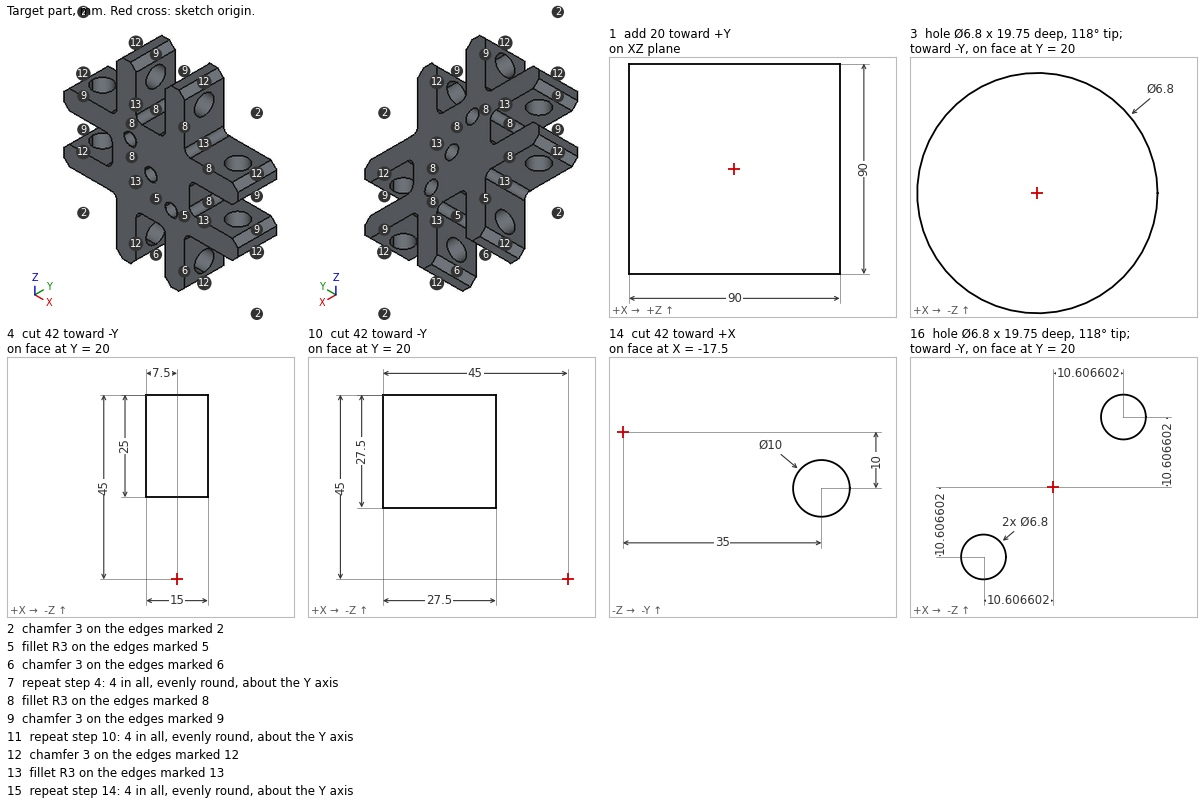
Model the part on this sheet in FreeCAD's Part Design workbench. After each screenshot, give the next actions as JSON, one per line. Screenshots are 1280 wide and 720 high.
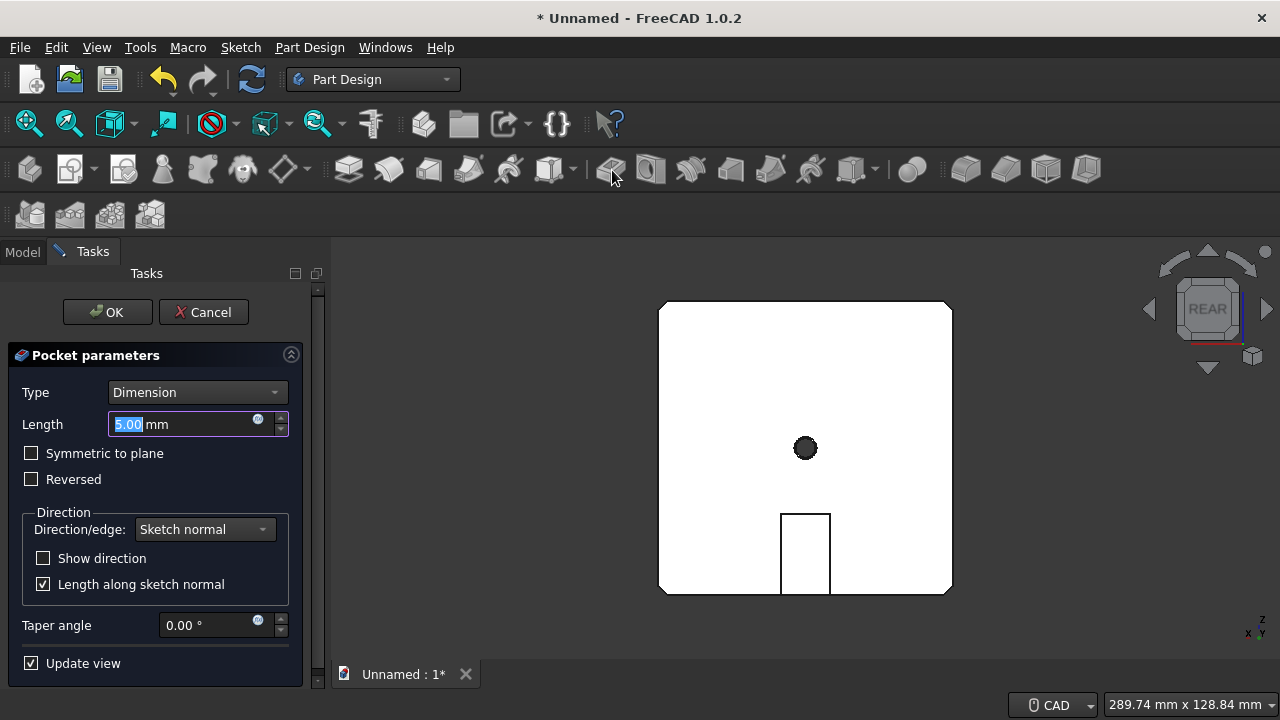
{"action": "type", "text": "42"}
{"action": "key", "text": "Tab"}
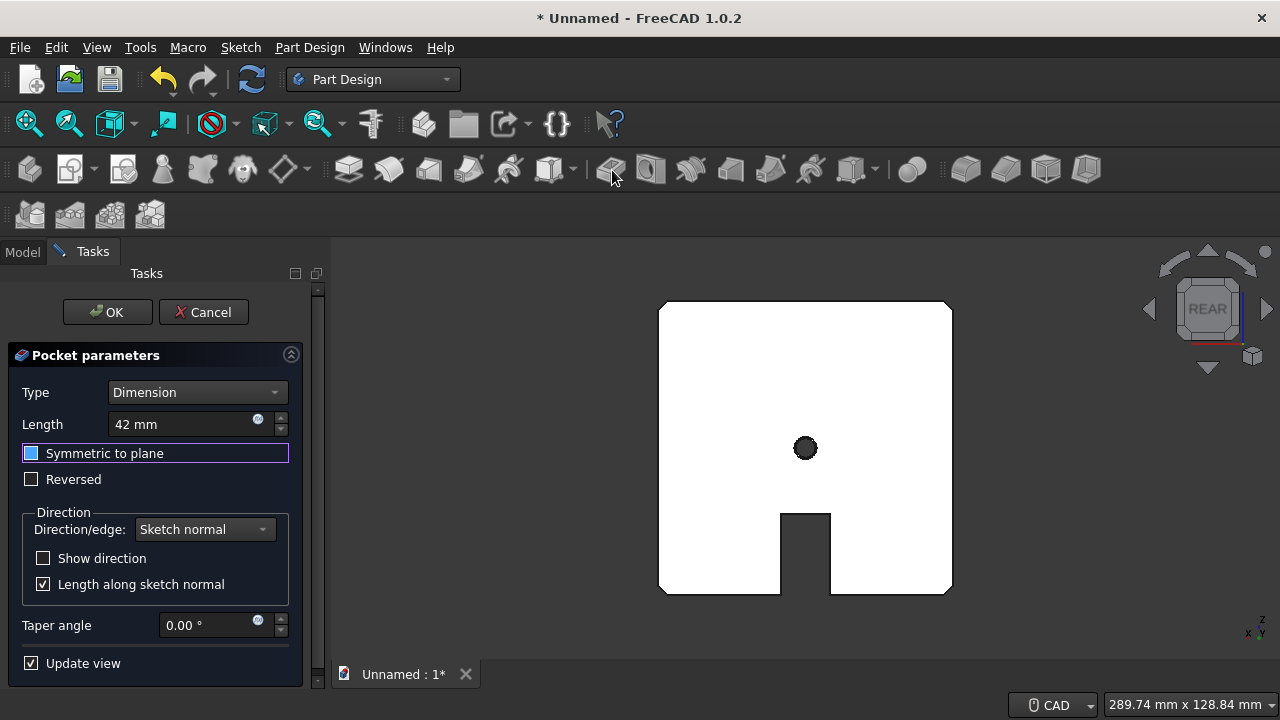
{"action": "left_click", "coordinate": [108, 312]}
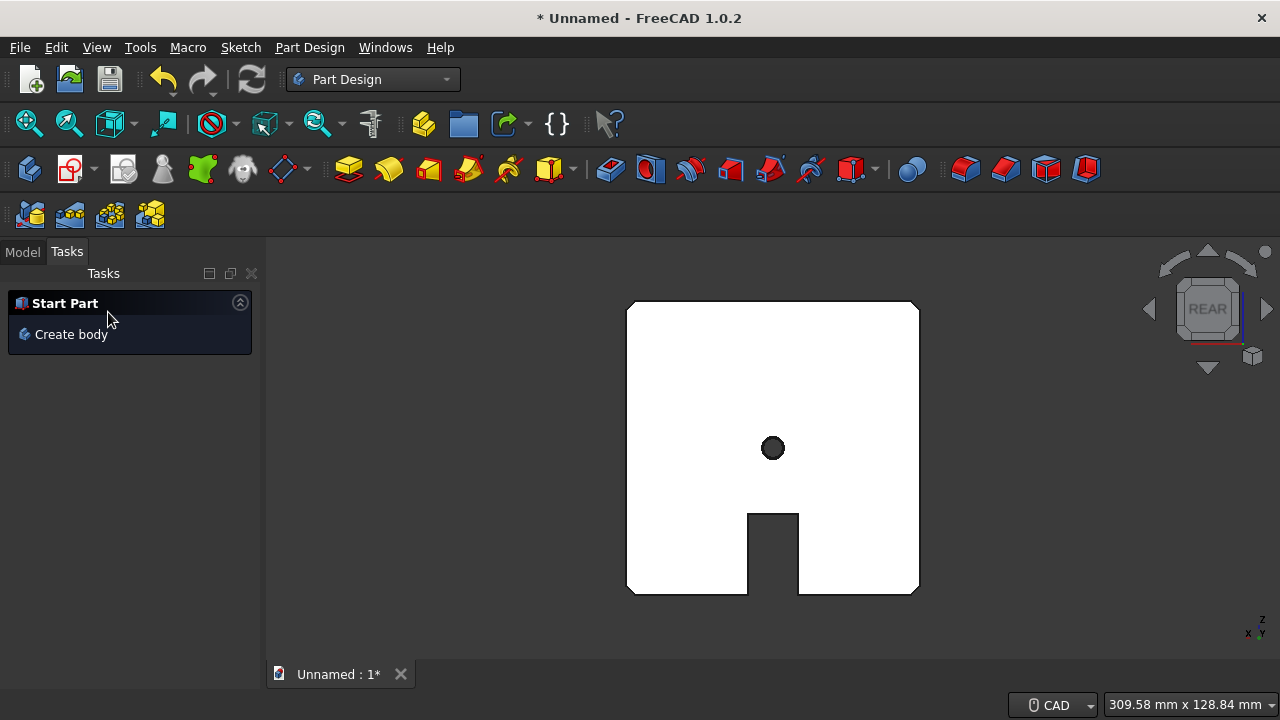
{"action": "key", "text": "0"}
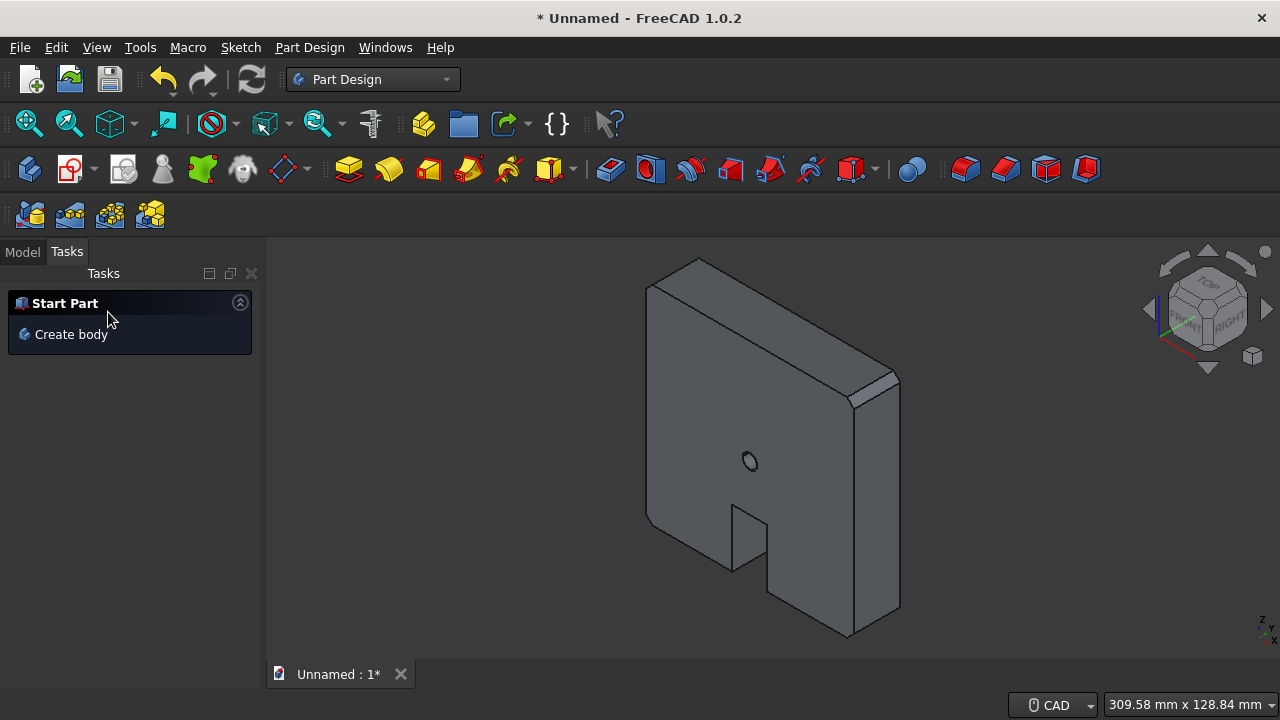
{"action": "key", "text": "2"}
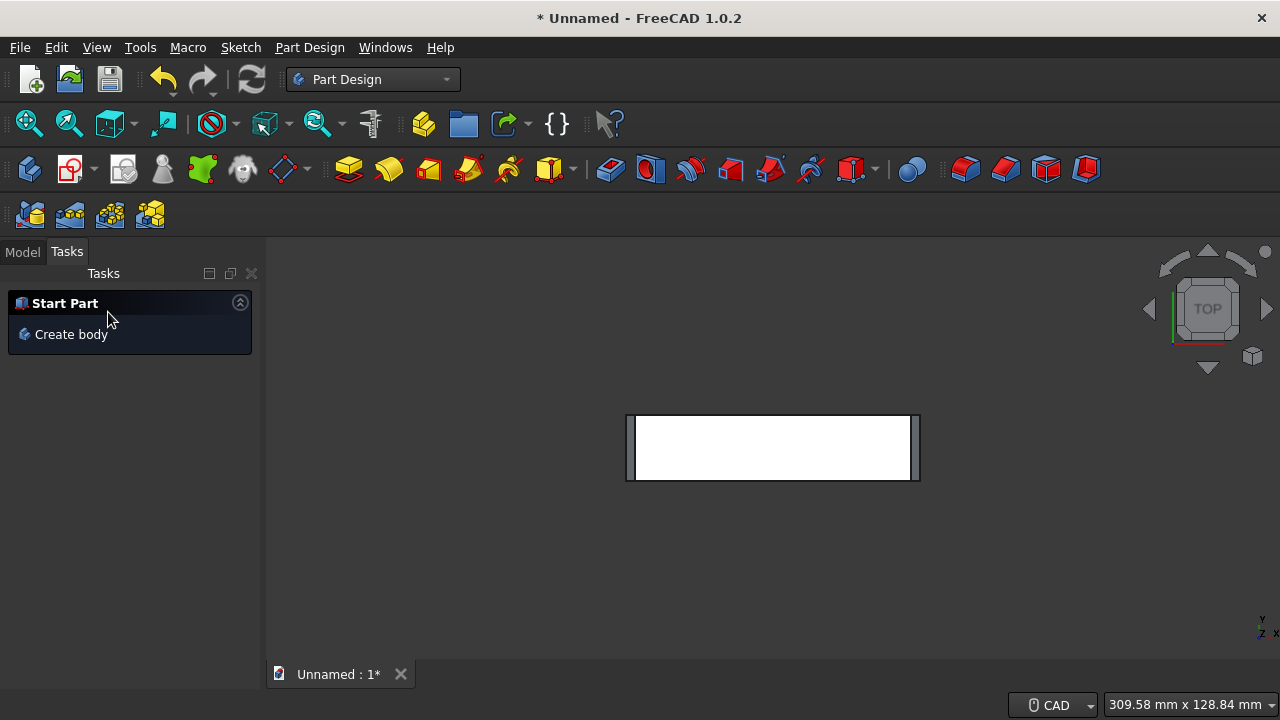
{"action": "left_click", "coordinate": [30, 124]}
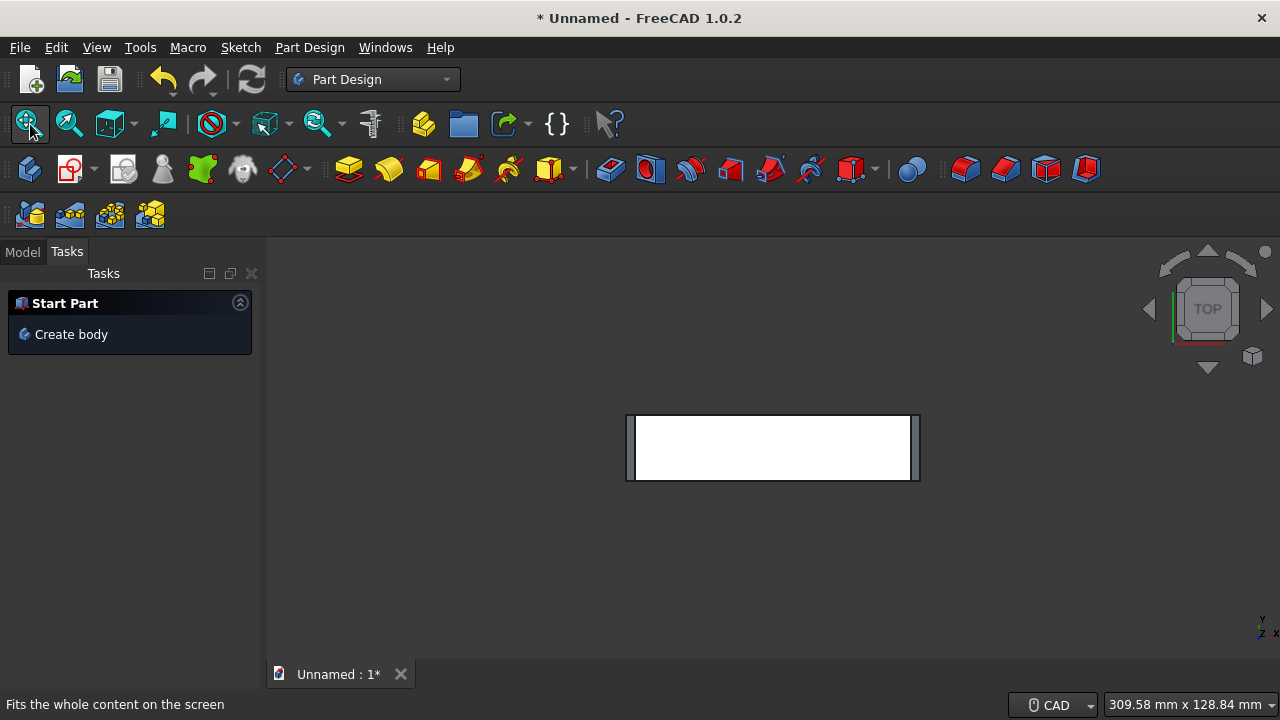
{"action": "key", "text": "1"}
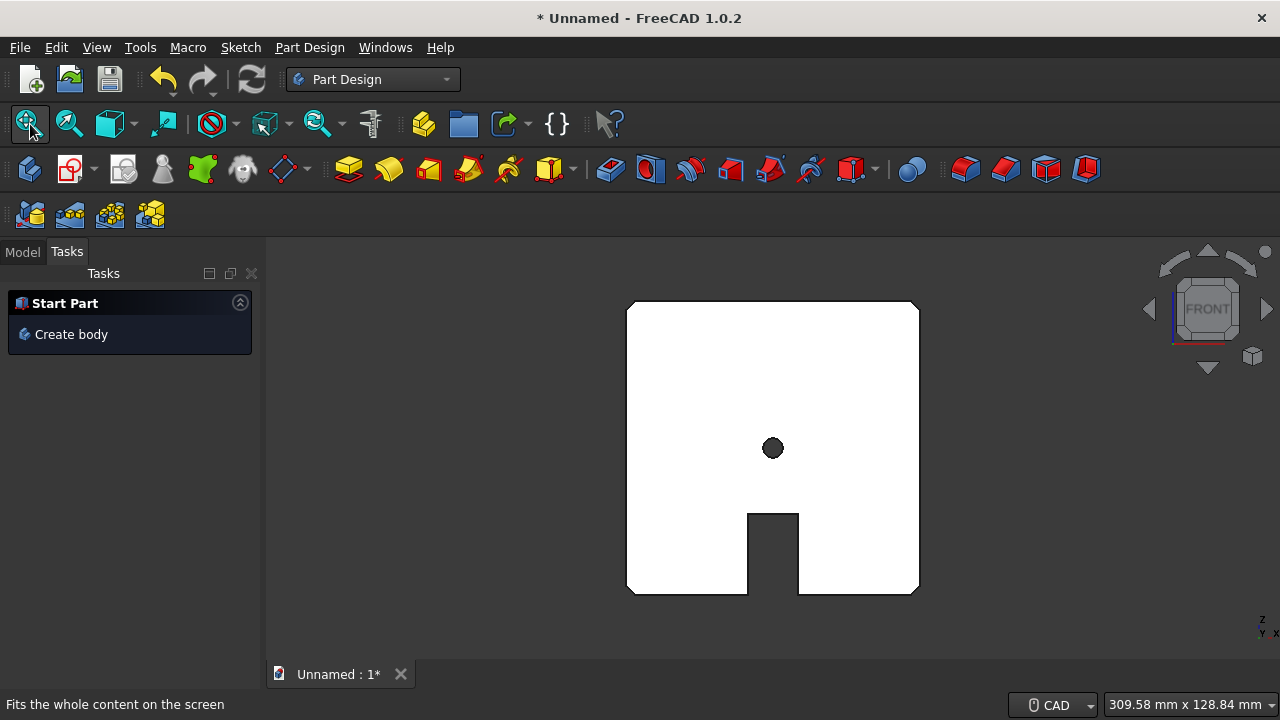
{"action": "key", "text": "3"}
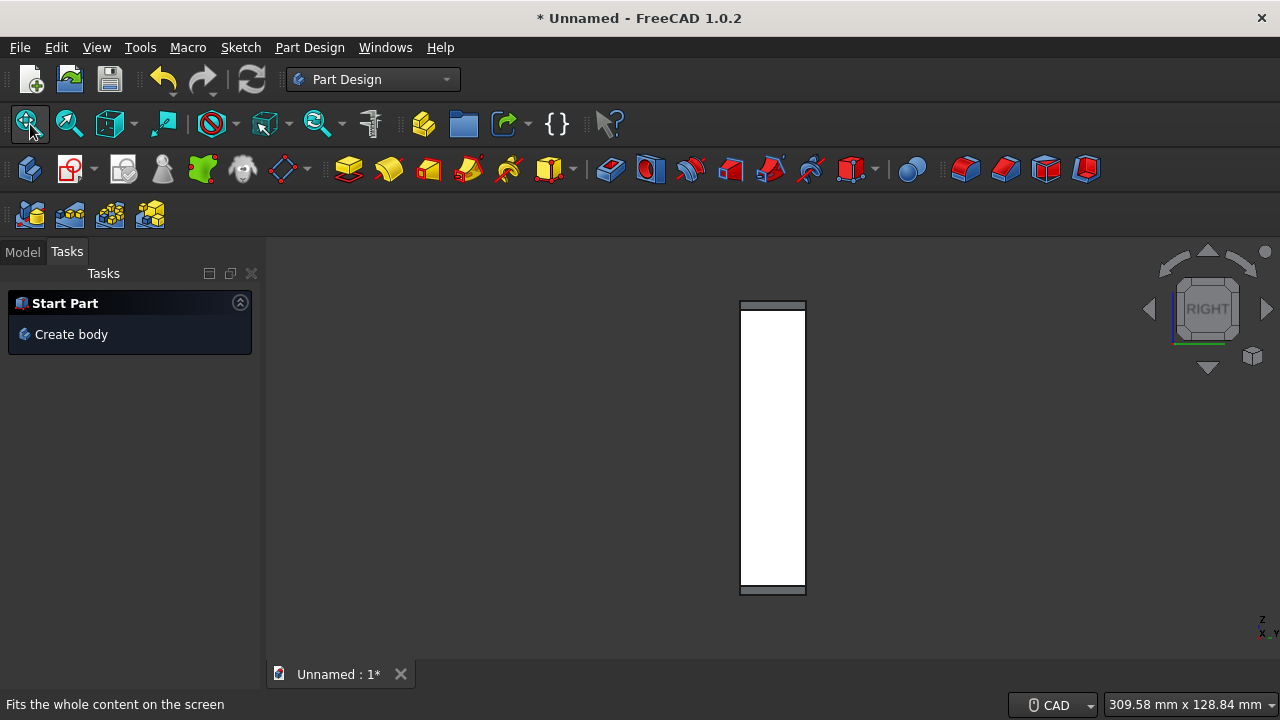
{"action": "key", "text": "5"}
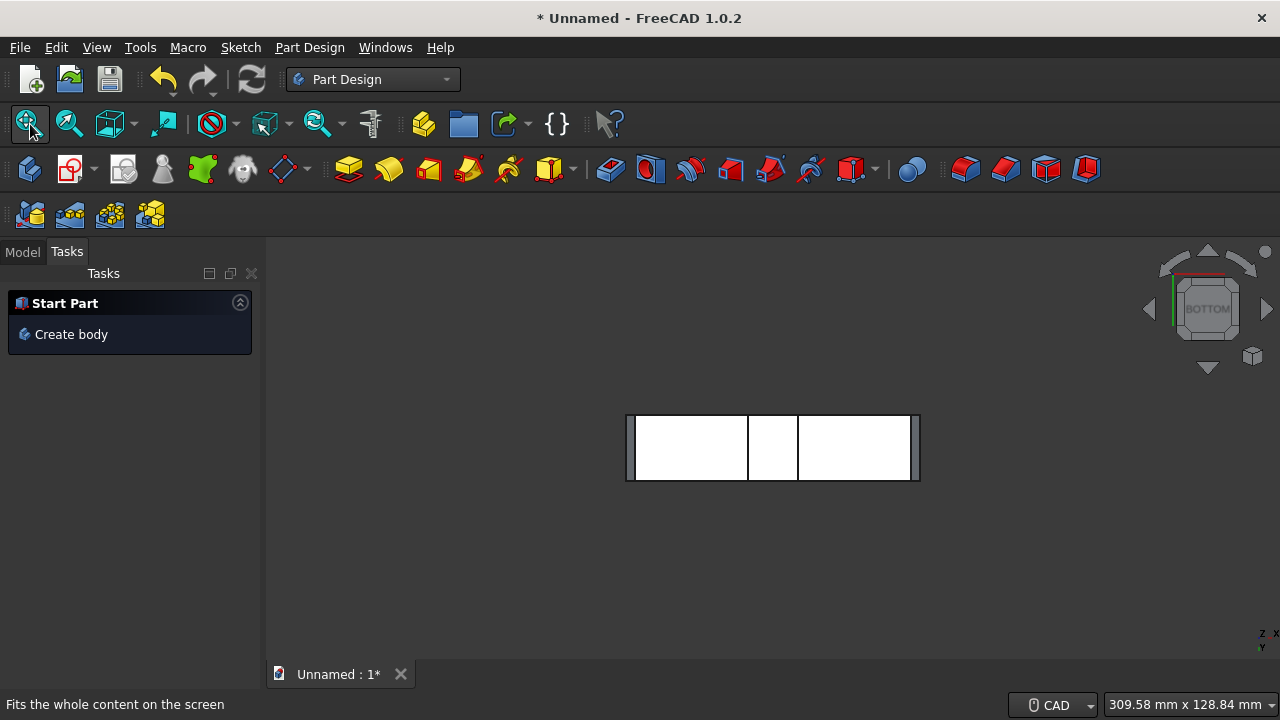
{"action": "left_click", "coordinate": [30, 124]}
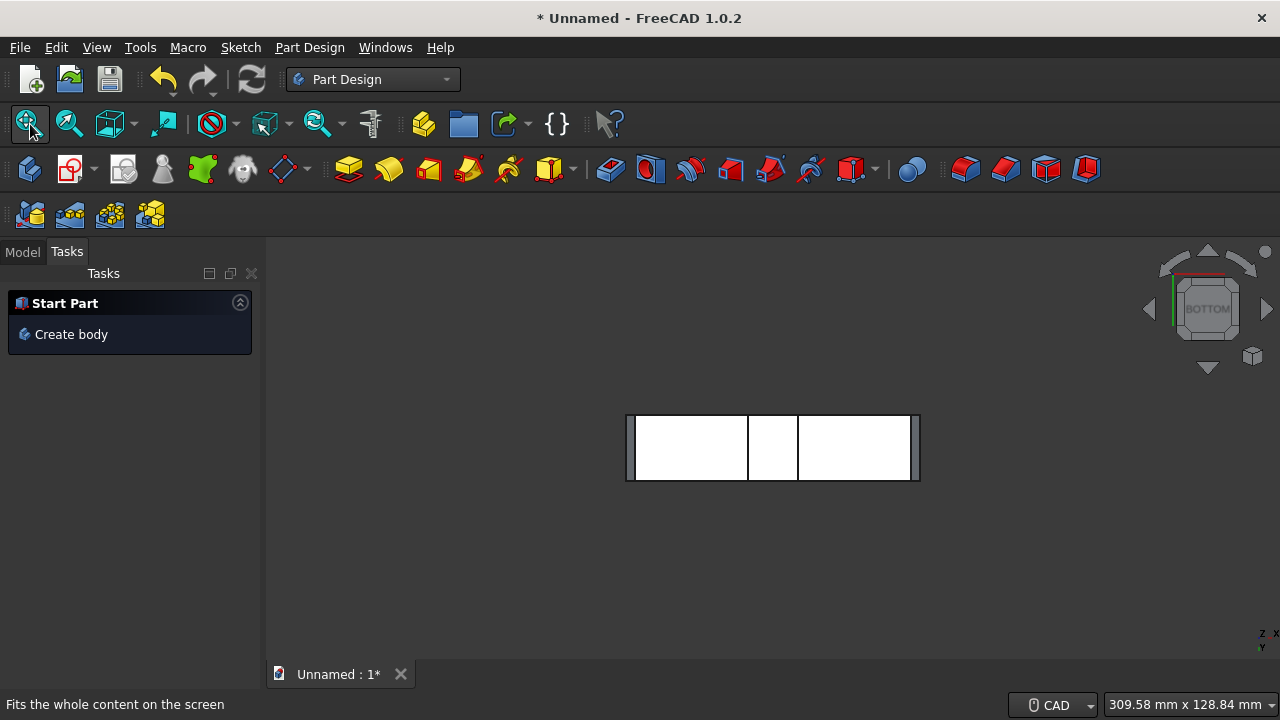
{"action": "key", "text": "4"}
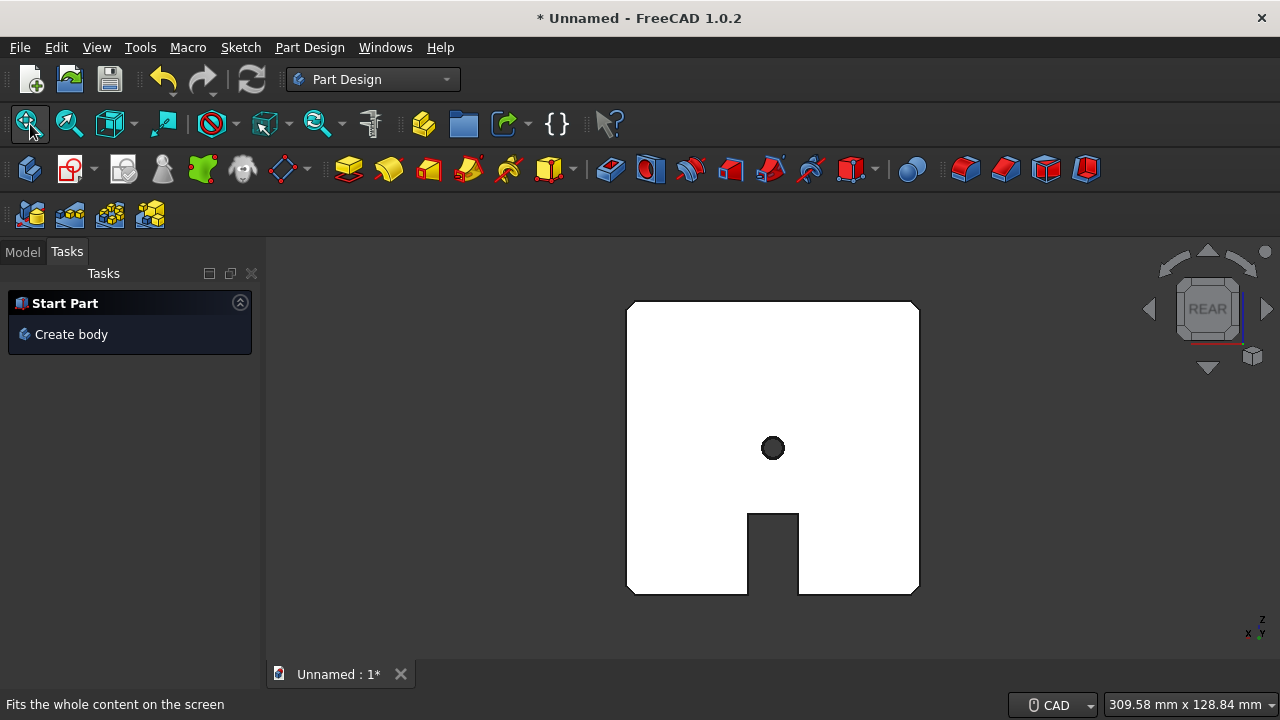
{"action": "key", "text": "6"}